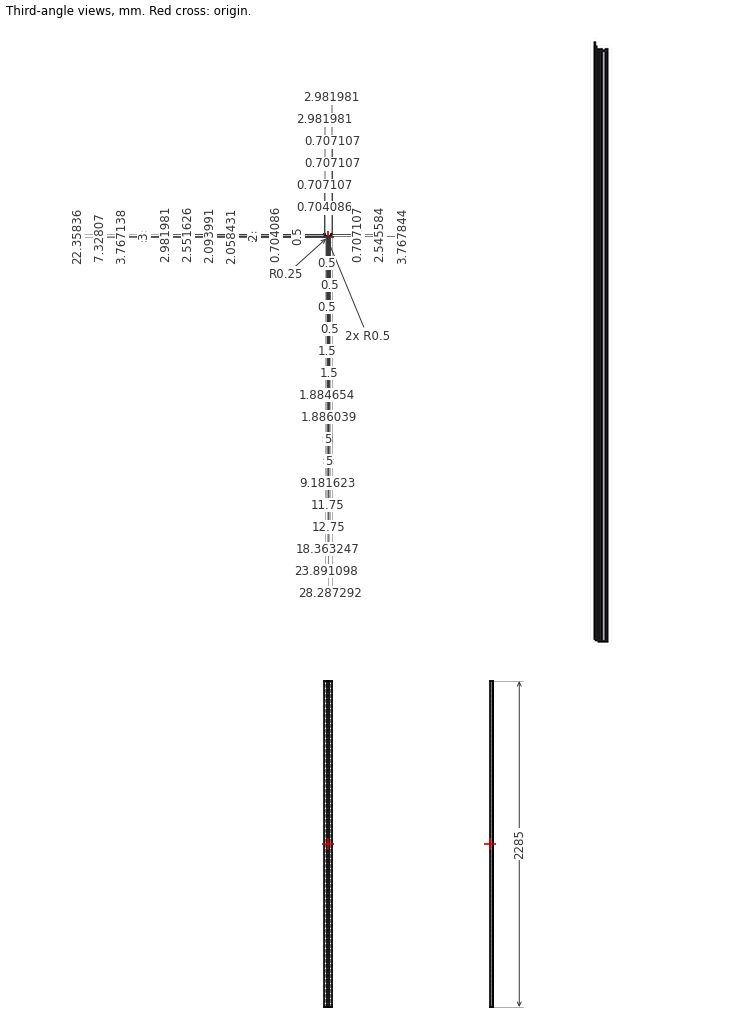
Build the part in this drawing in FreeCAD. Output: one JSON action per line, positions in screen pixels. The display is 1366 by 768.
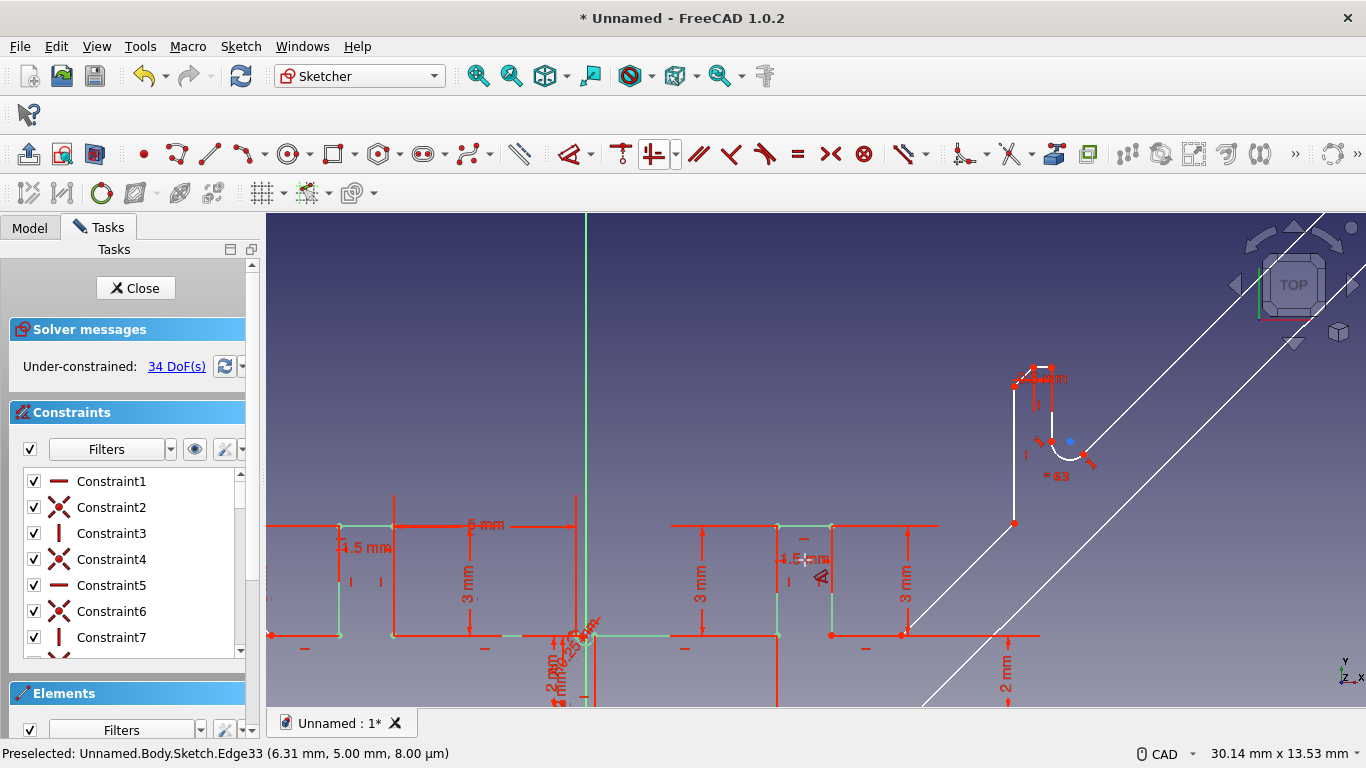
{"action": "scroll", "coordinate": [817, 529], "scroll_direction": "down", "scroll_amount": 6}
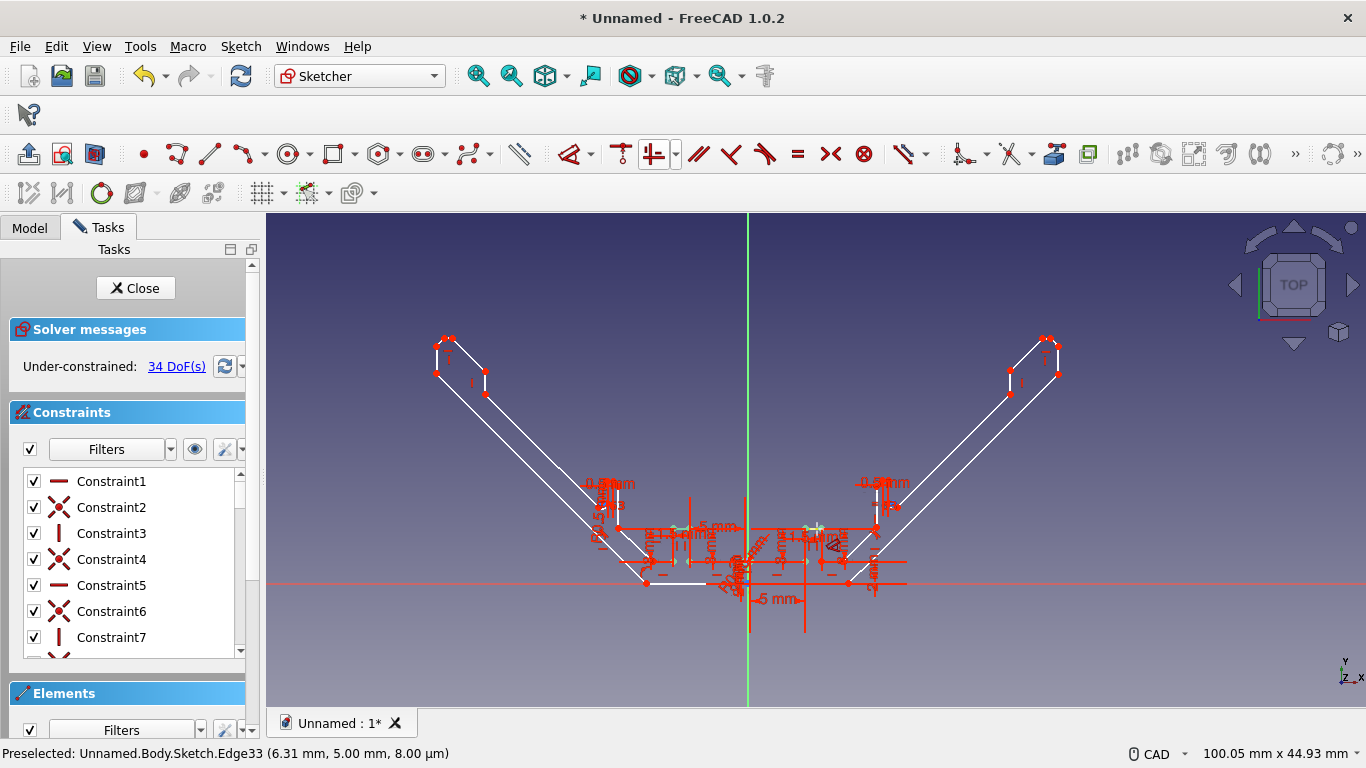
{"action": "scroll", "coordinate": [616, 485], "scroll_direction": "up", "scroll_amount": 10}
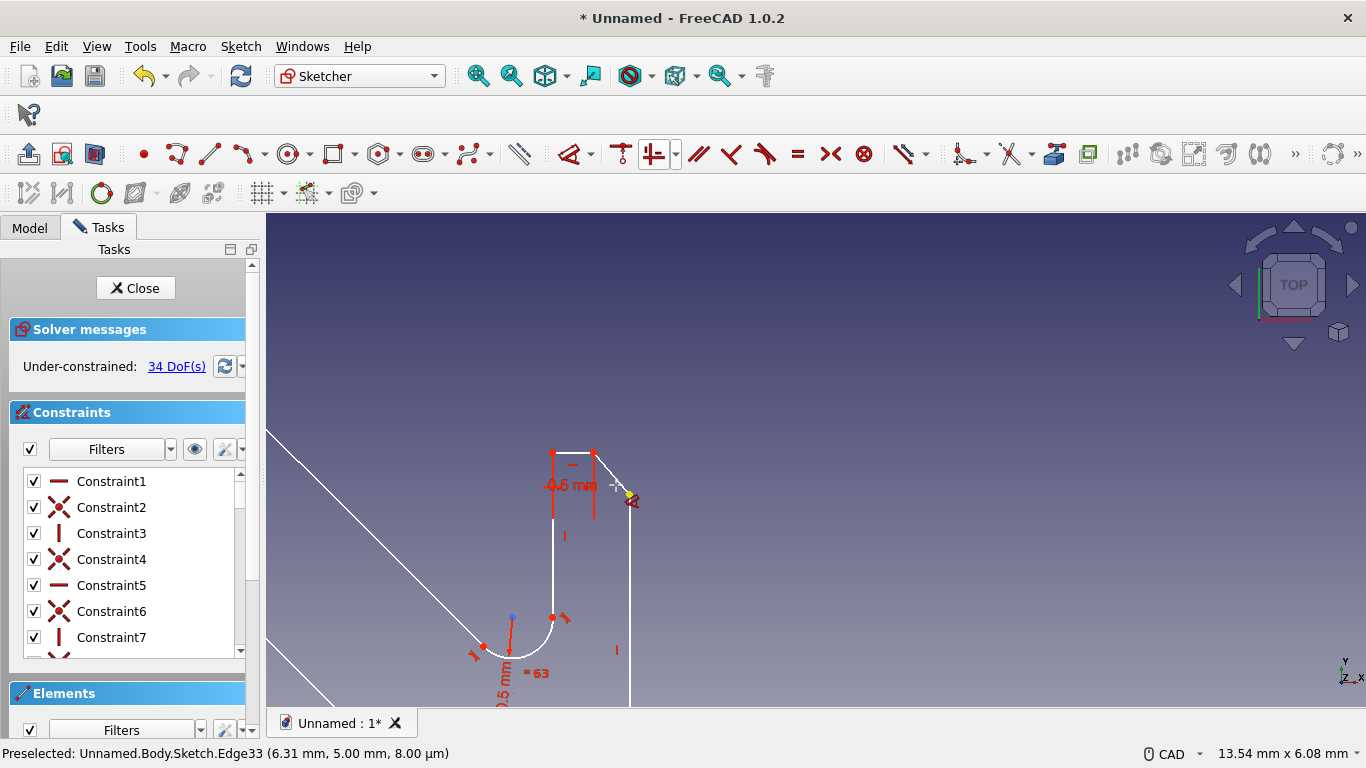
{"action": "left_click", "coordinate": [615, 478]}
{"action": "left_click", "coordinate": [612, 529]}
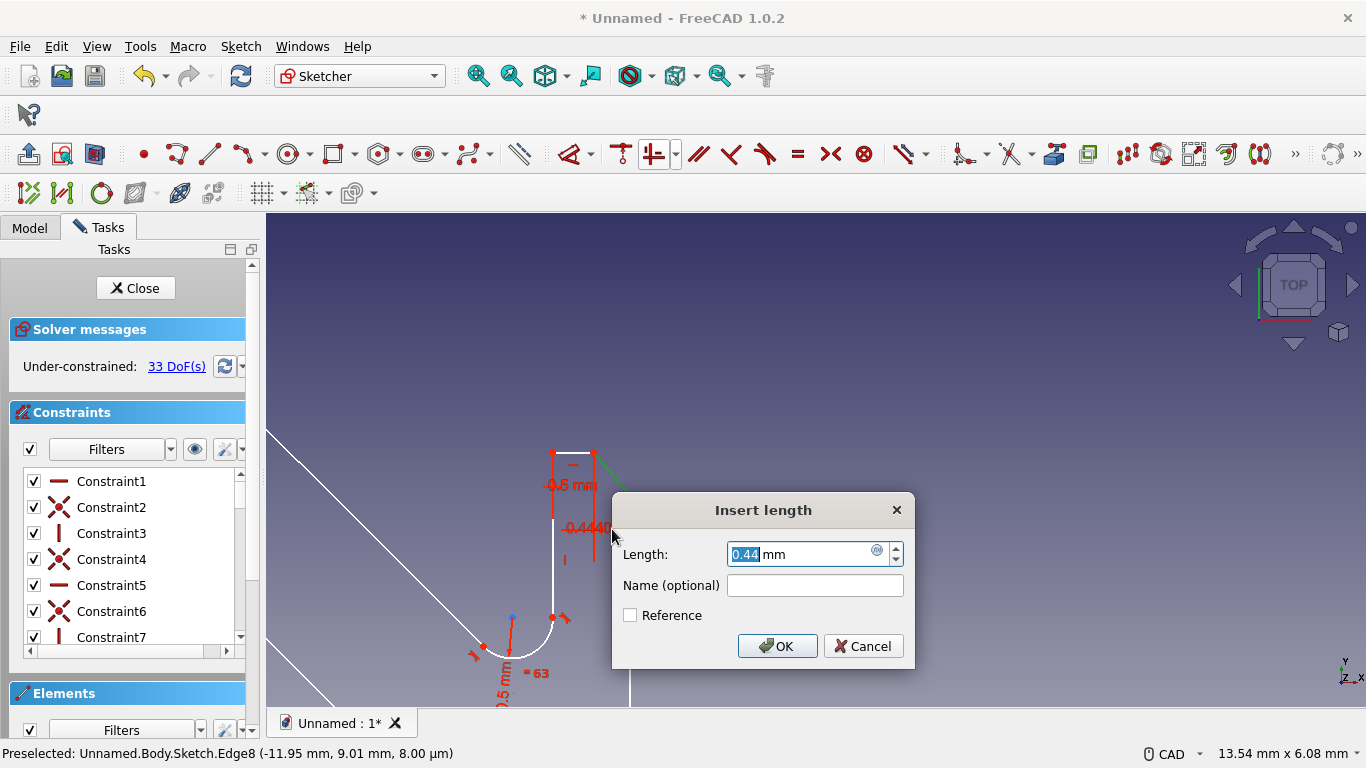
{"action": "type", "text": "0.5"}
{"action": "key", "text": "Return"}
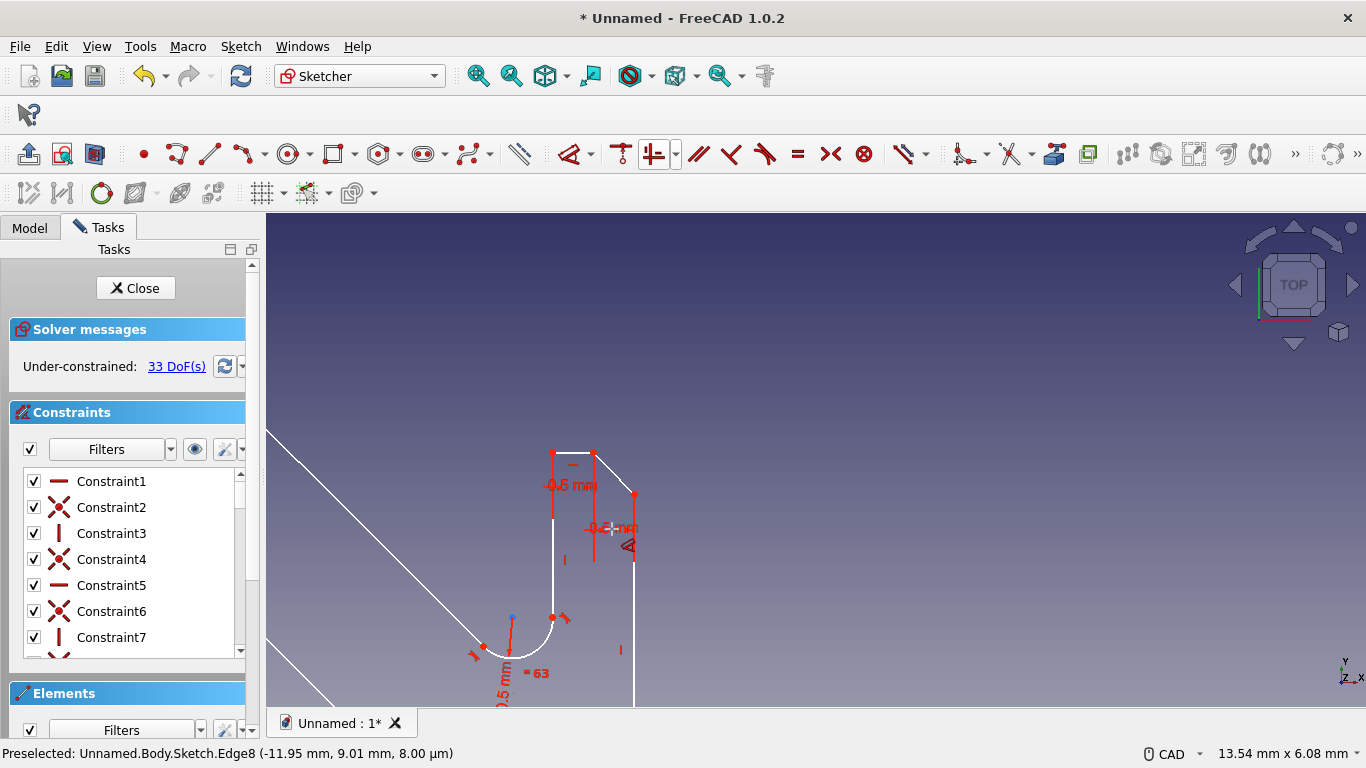
{"action": "left_click", "coordinate": [622, 482]}
{"action": "left_click", "coordinate": [668, 474]}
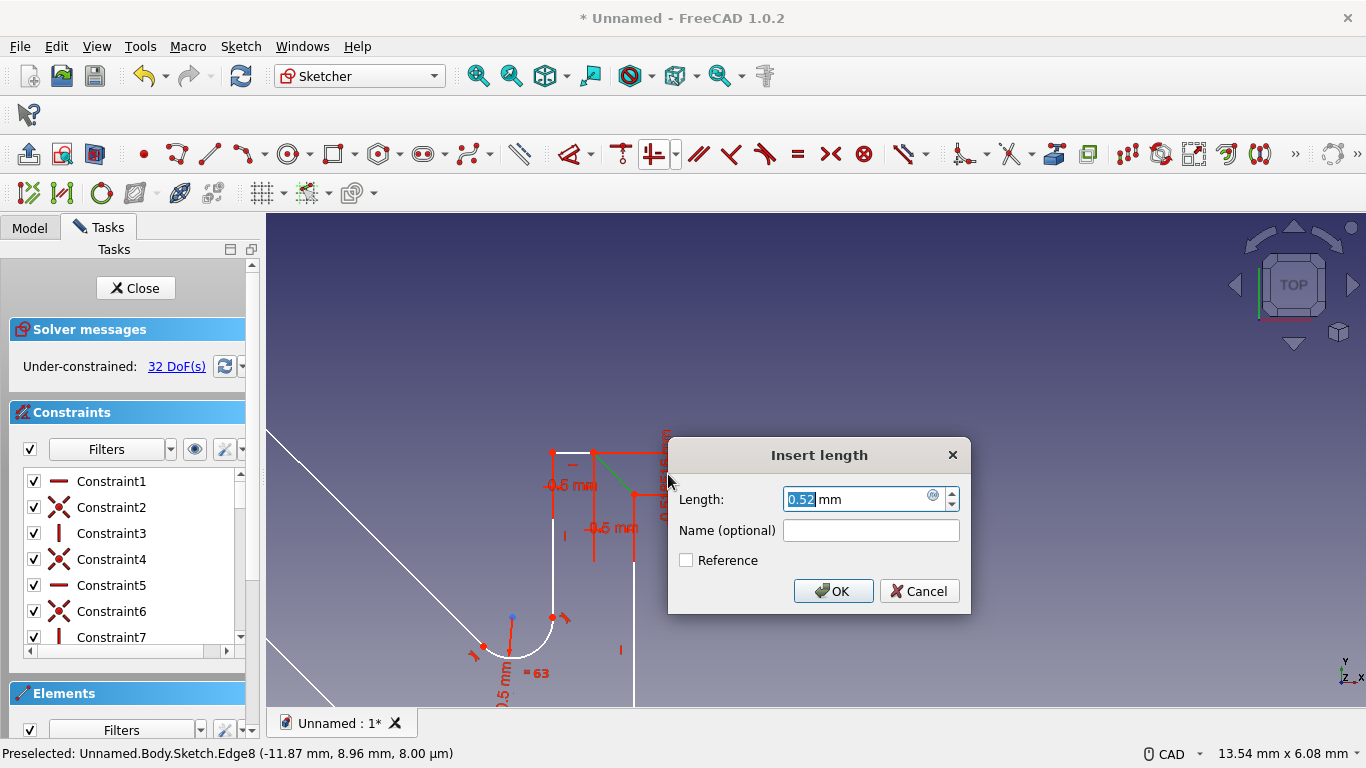
{"action": "type", "text": "0.5"}
{"action": "key", "text": "Return"}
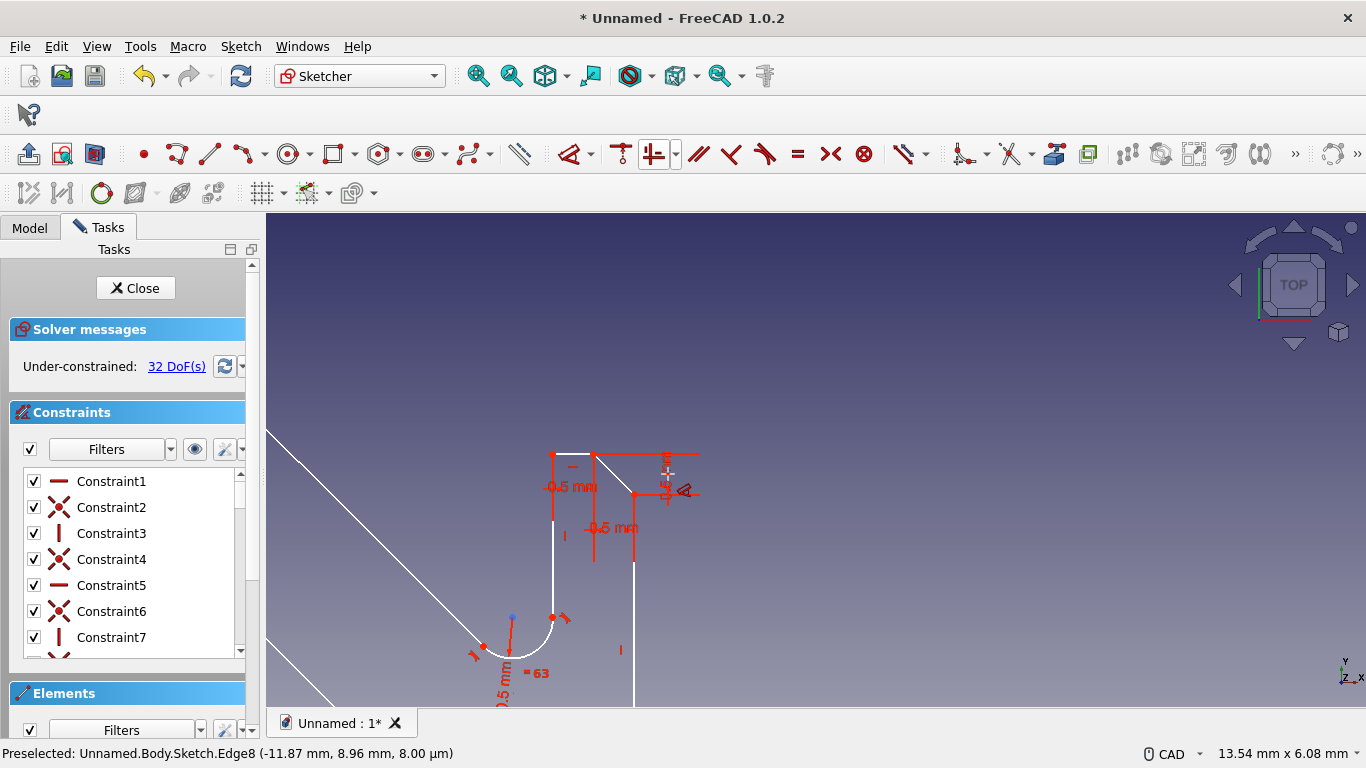
{"action": "scroll", "coordinate": [616, 485], "scroll_direction": "down", "scroll_amount": 10}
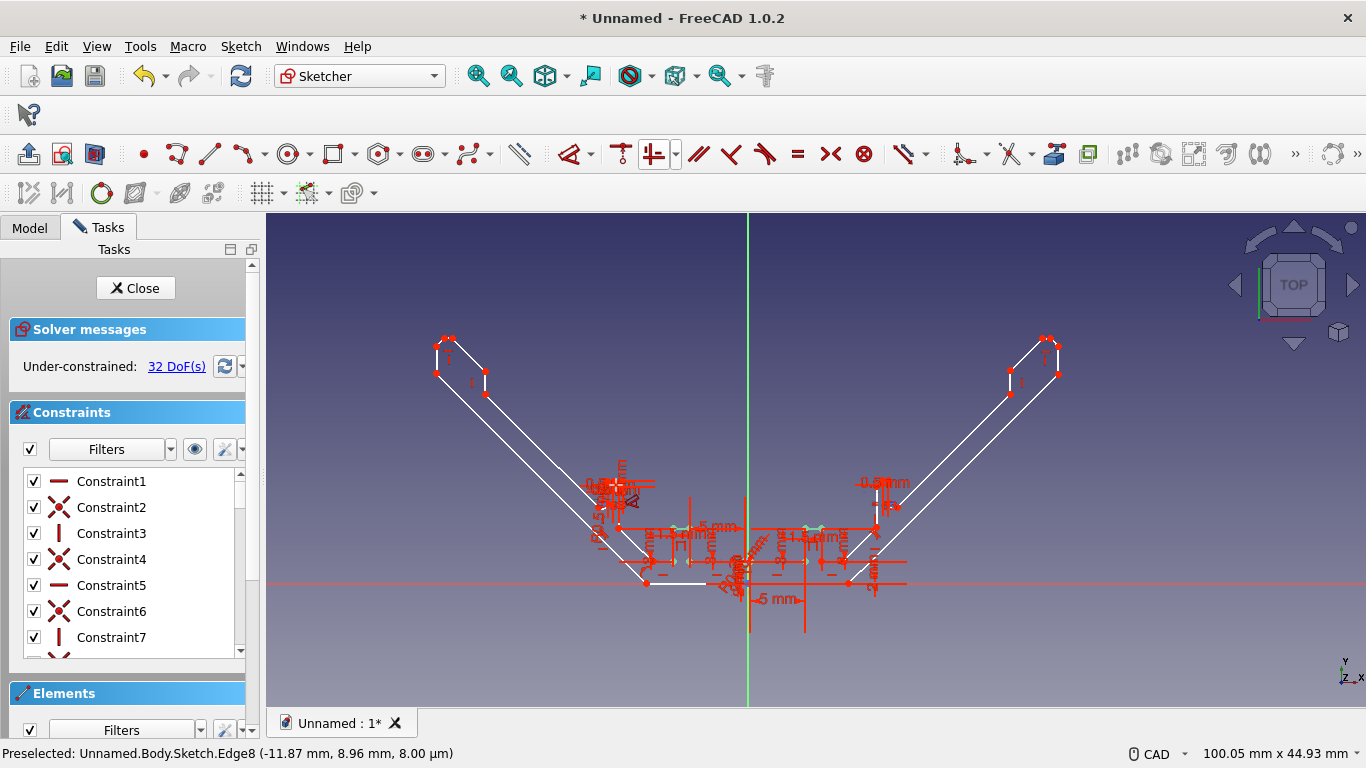
{"action": "scroll", "coordinate": [881, 482], "scroll_direction": "up", "scroll_amount": 10}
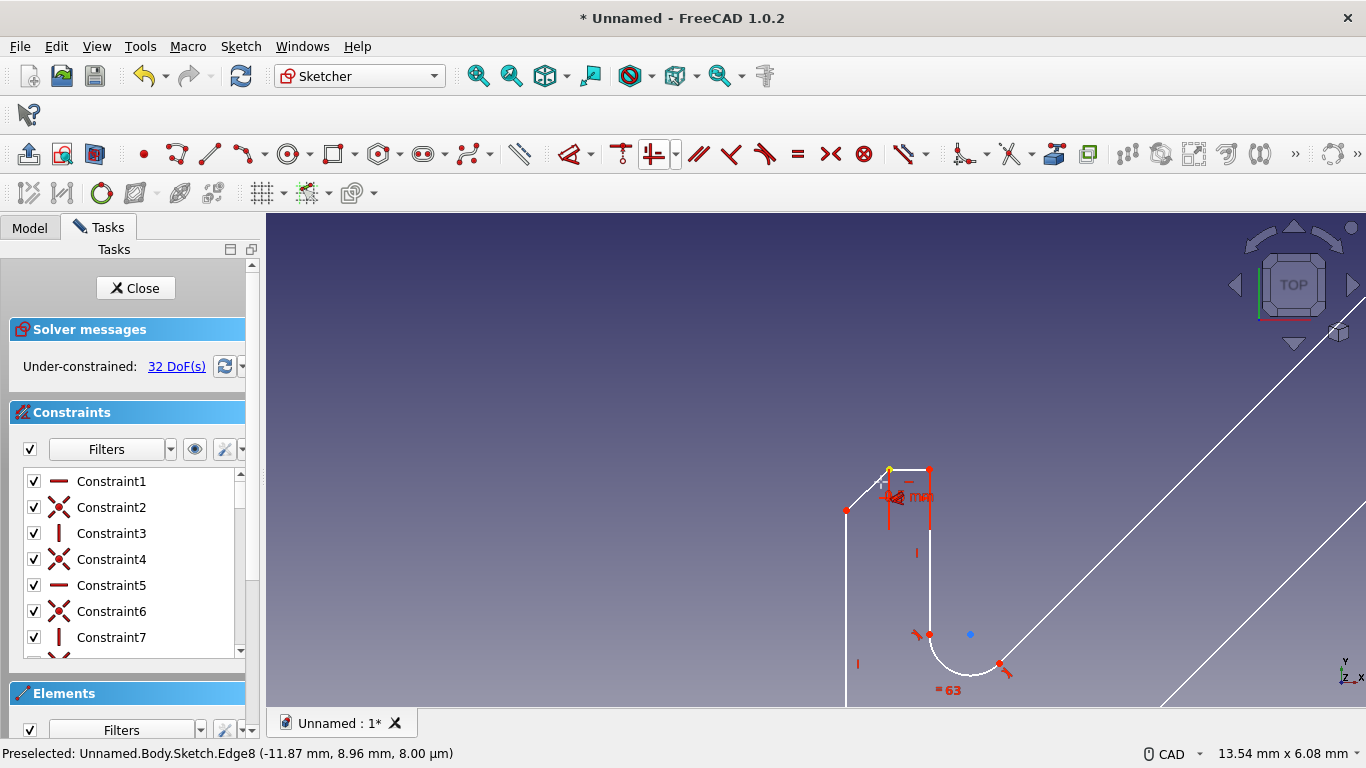
{"action": "left_click", "coordinate": [876, 482]}
{"action": "left_click", "coordinate": [868, 545]}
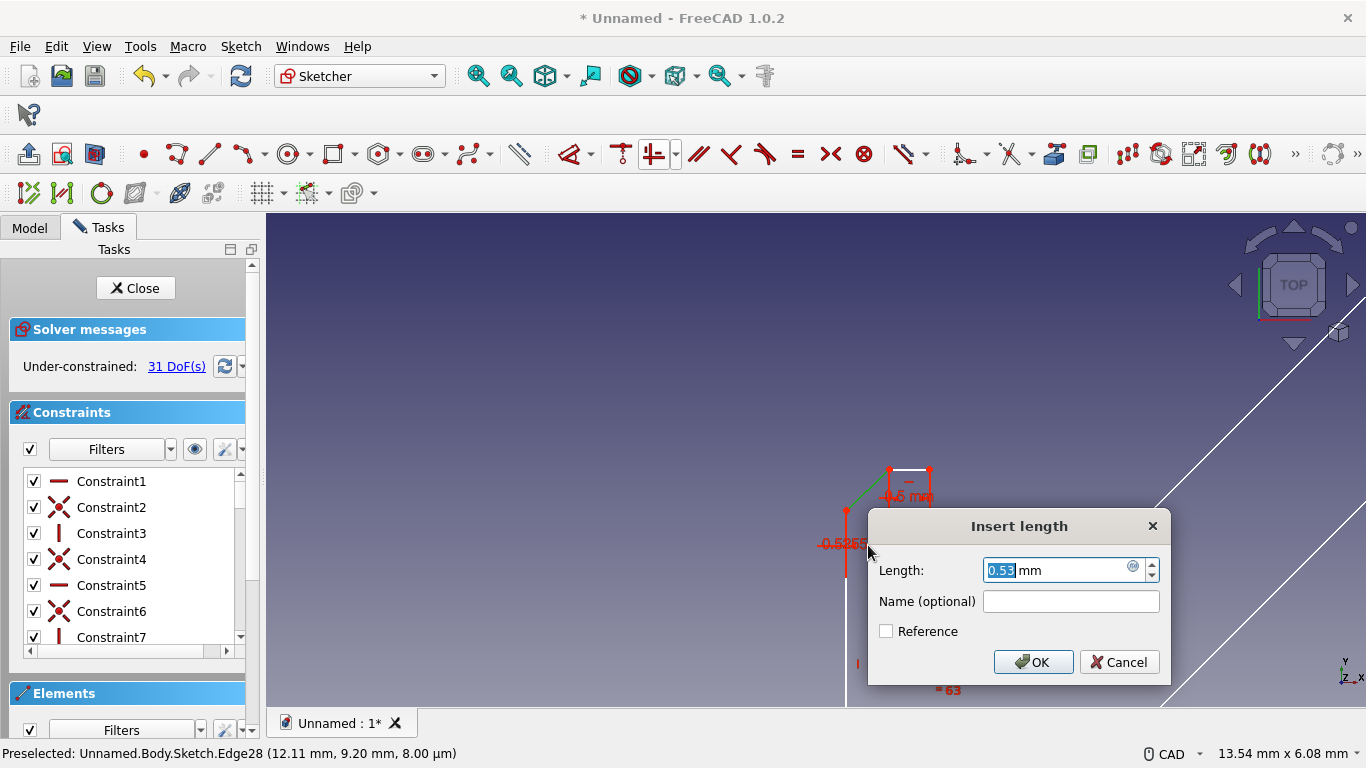
{"action": "type", "text": "0.5"}
{"action": "key", "text": "Return"}